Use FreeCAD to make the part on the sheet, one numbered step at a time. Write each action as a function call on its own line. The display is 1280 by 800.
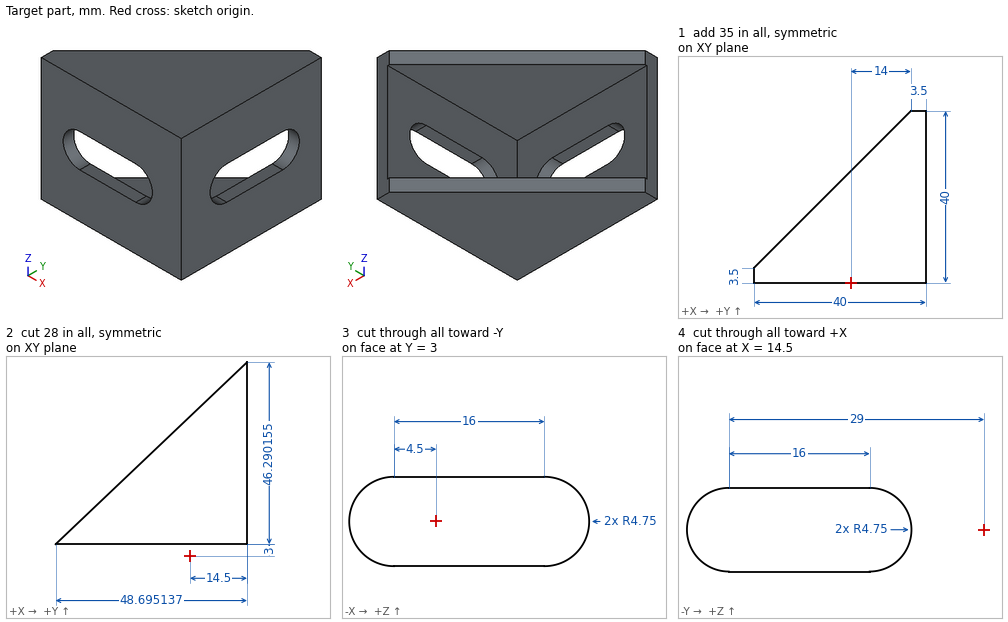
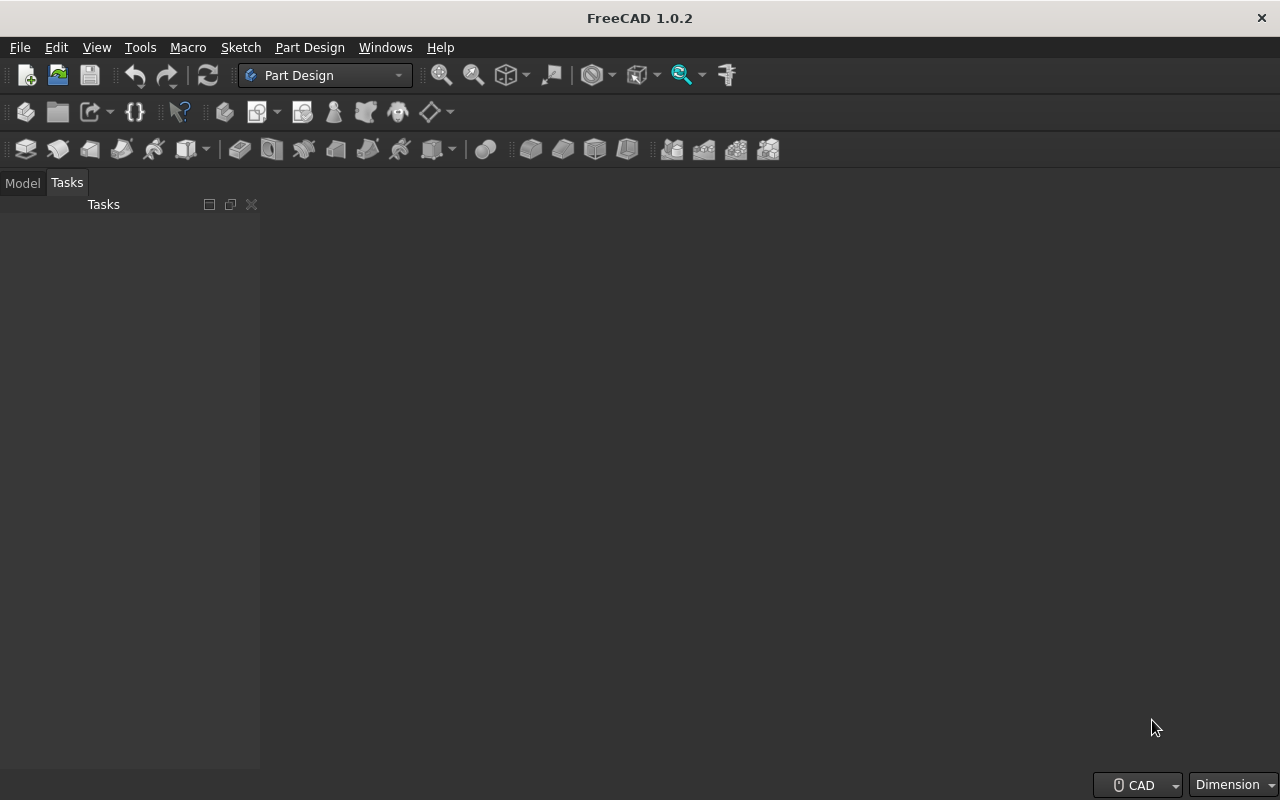
click(26, 76)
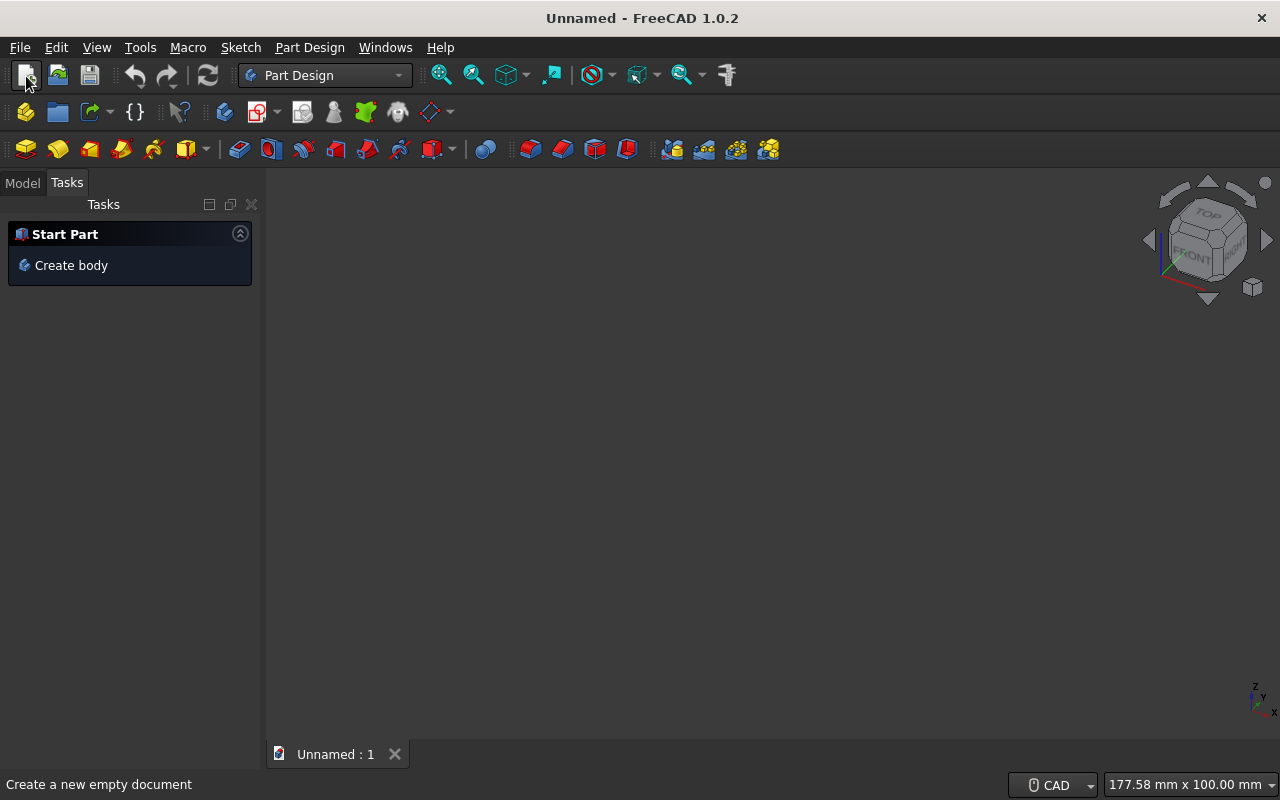
click(258, 112)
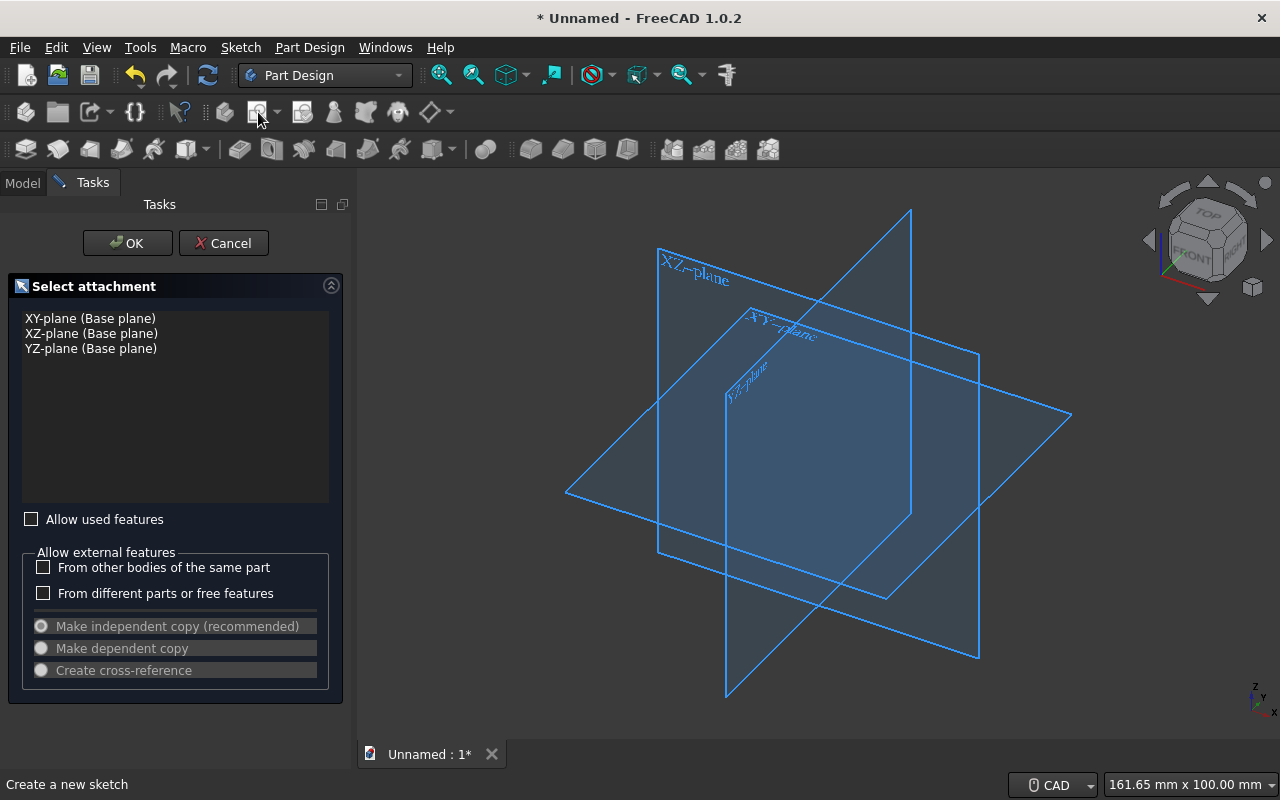
click(82, 318)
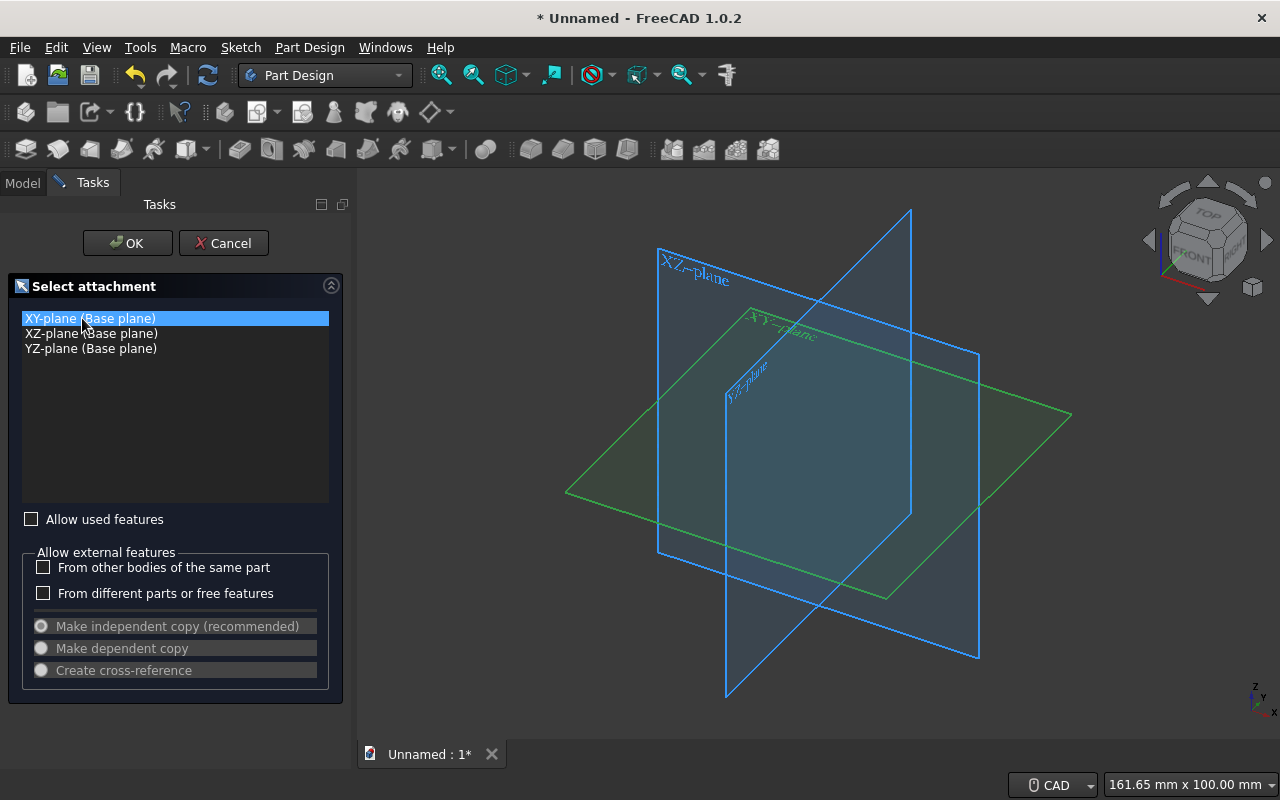
click(128, 243)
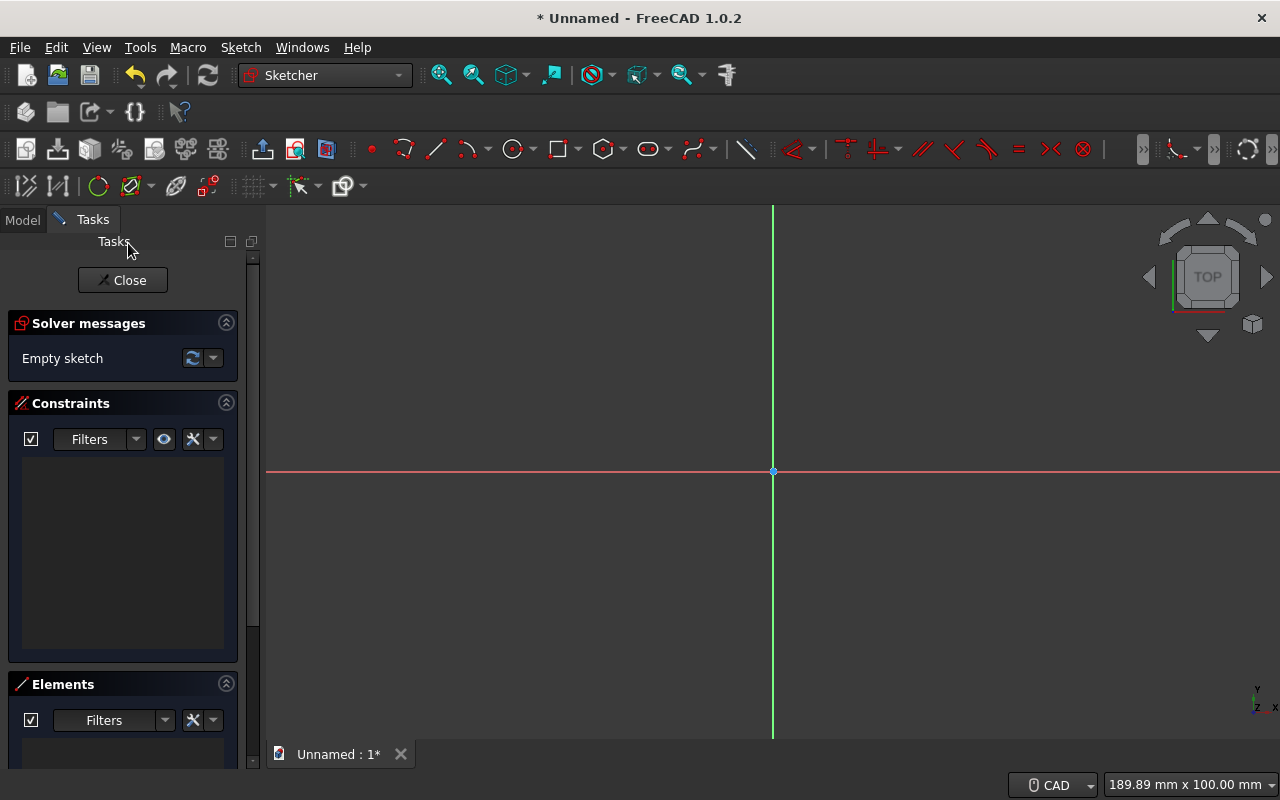
scroll(872, 233, up, 2)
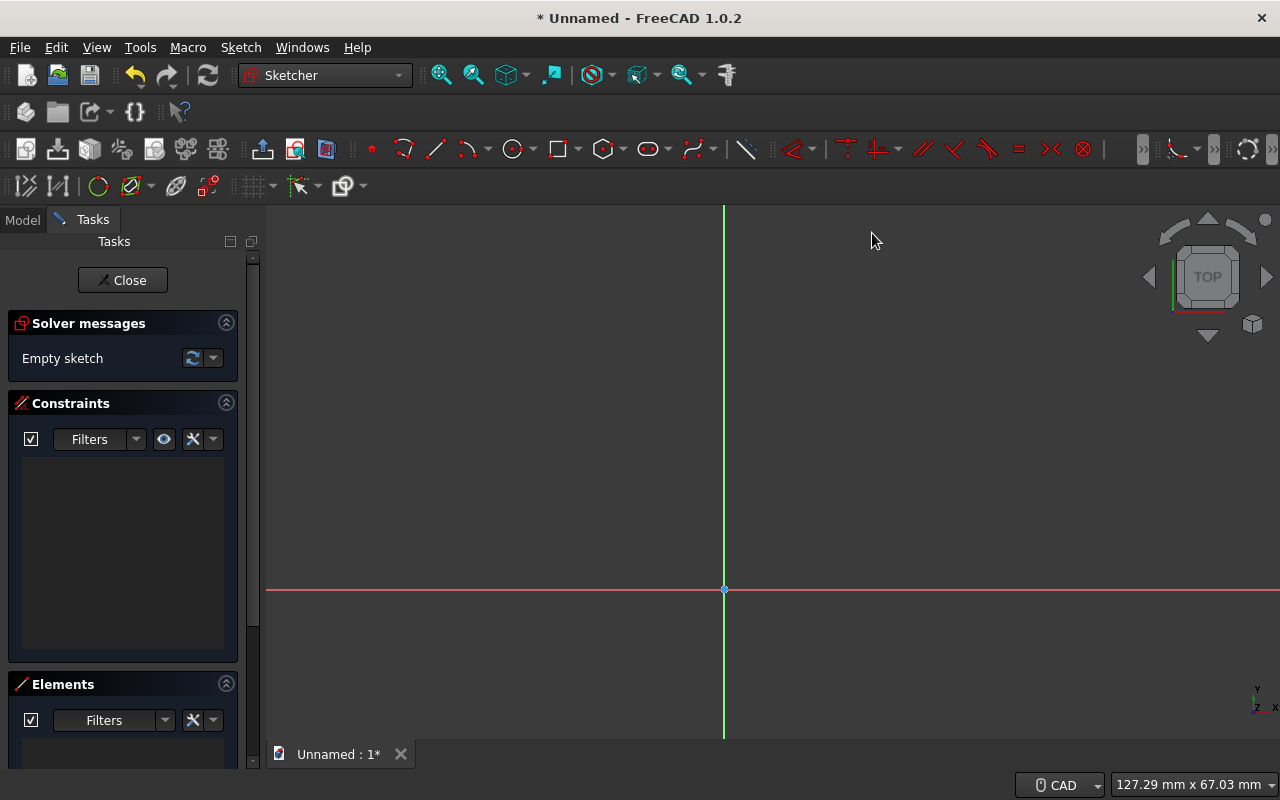
click(404, 150)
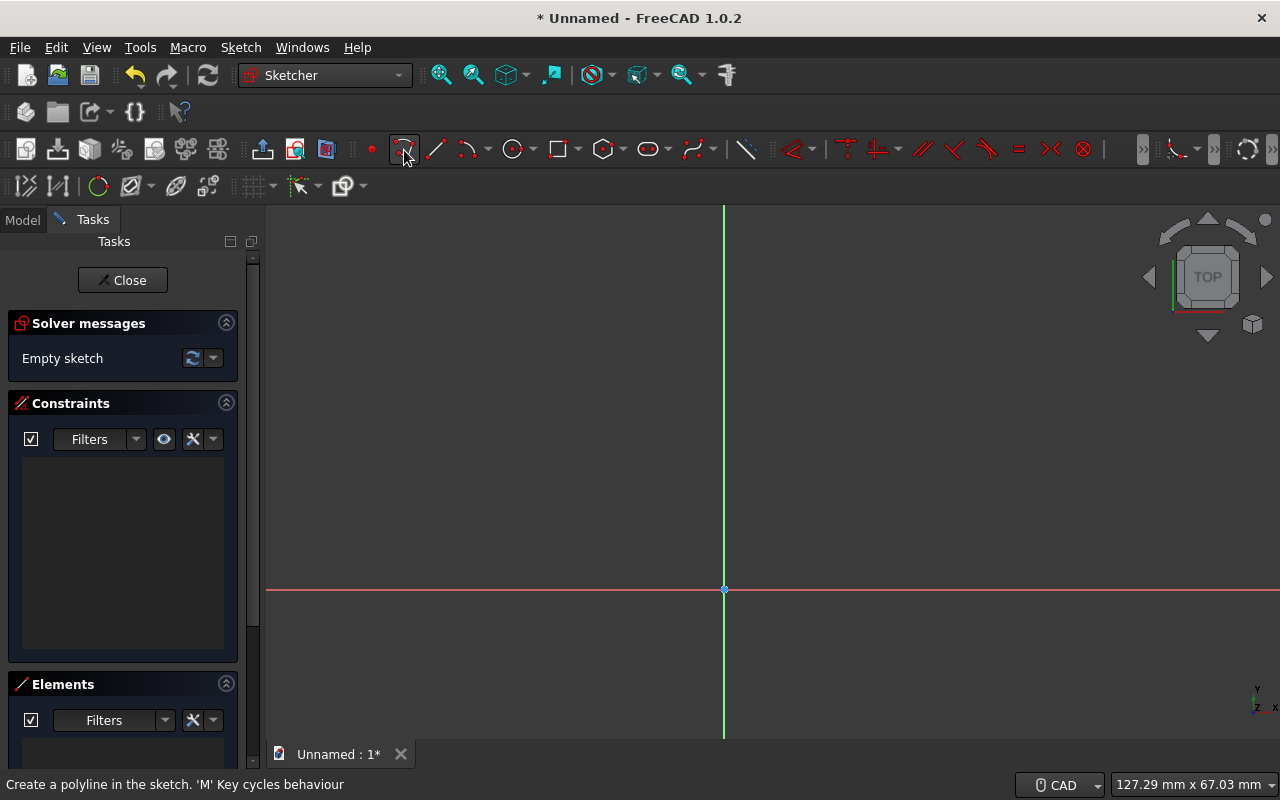
click(863, 590)
click(863, 271)
click(836, 271)
click(545, 562)
click(545, 581)
click(863, 590)
key(Escape)
key(Escape)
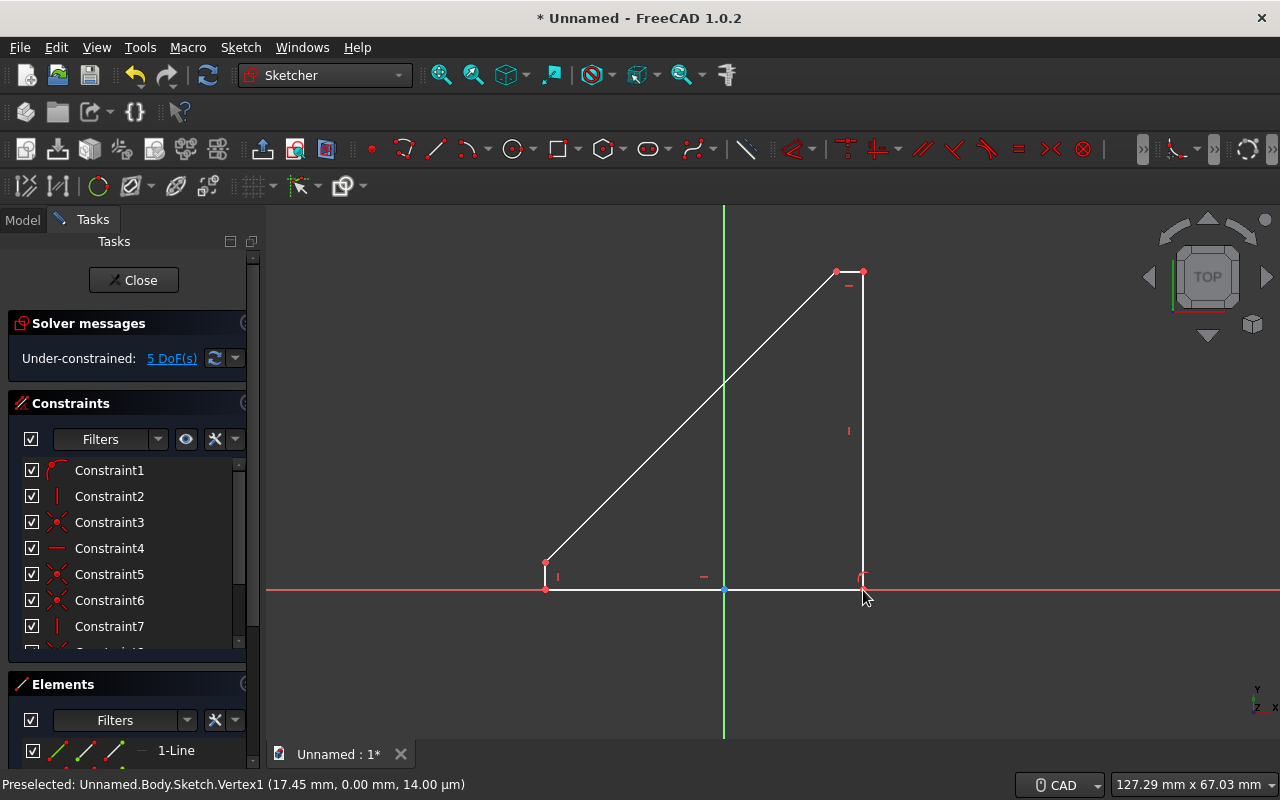
click(863, 494)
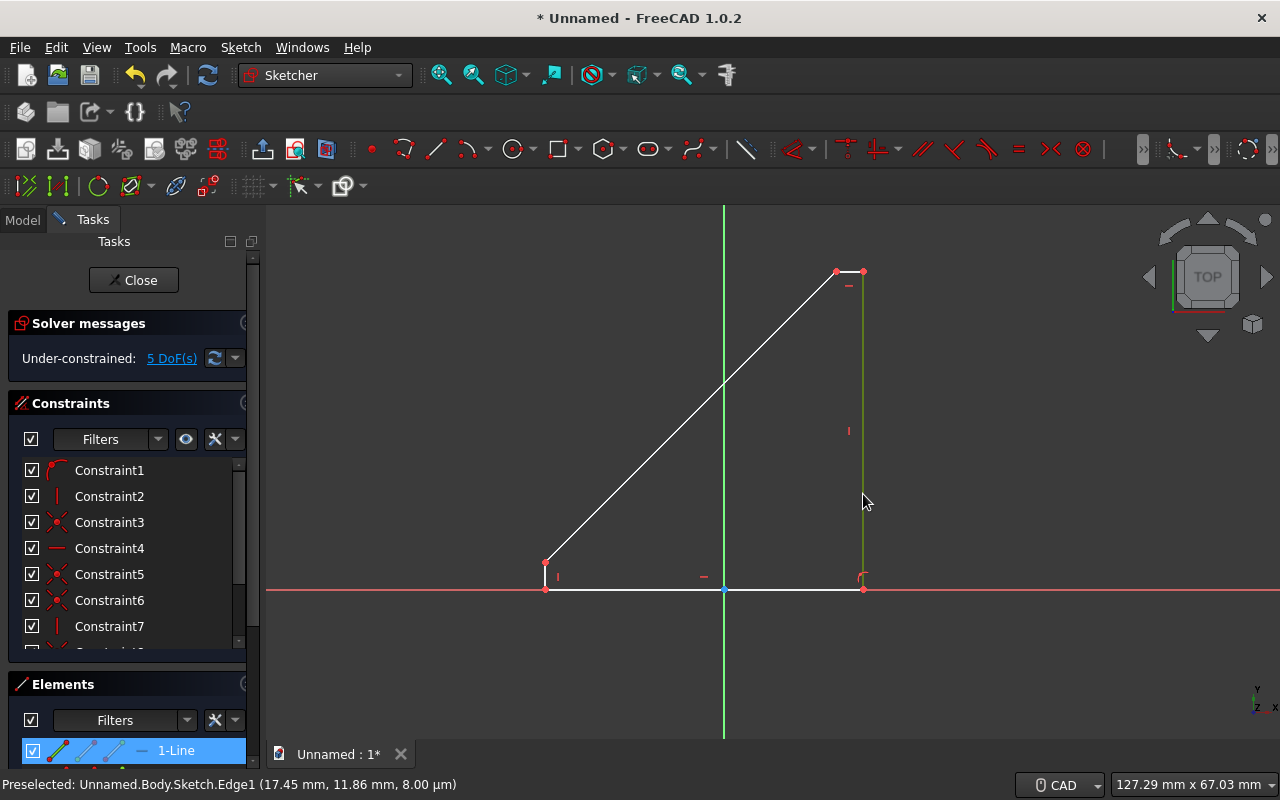
key(i)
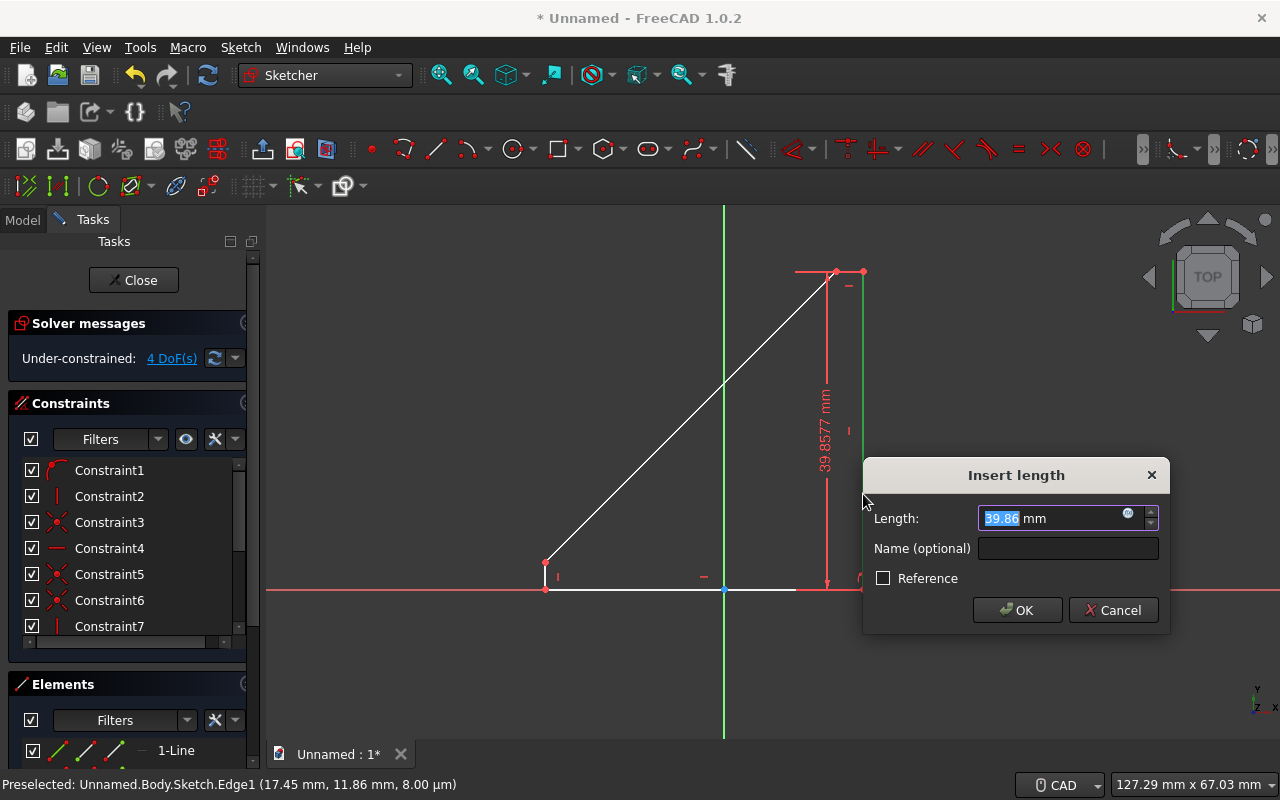
text(40)
key(Return)